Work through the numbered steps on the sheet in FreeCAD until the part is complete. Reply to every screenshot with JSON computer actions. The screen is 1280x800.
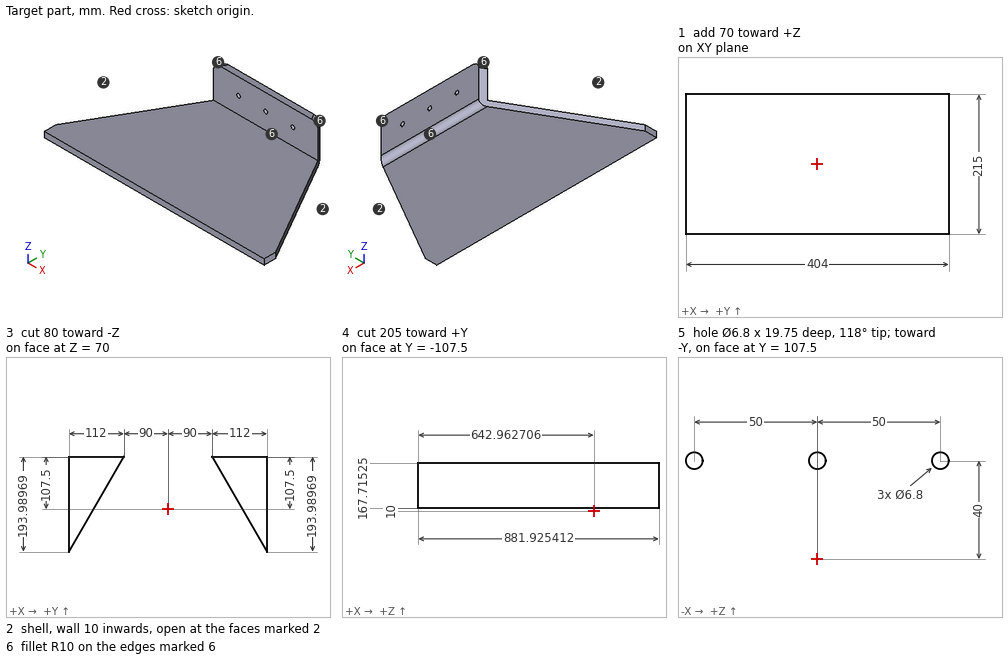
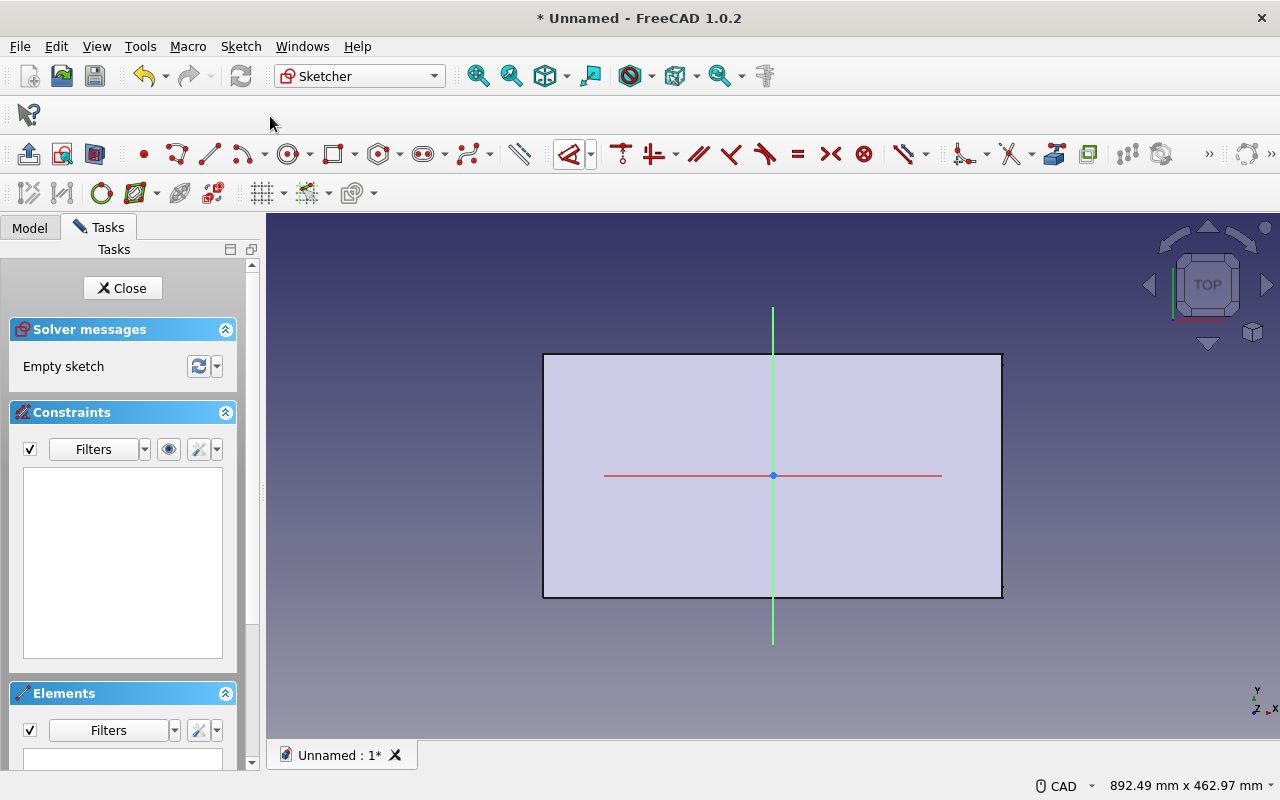
{"action": "left_click", "coordinate": [177, 154]}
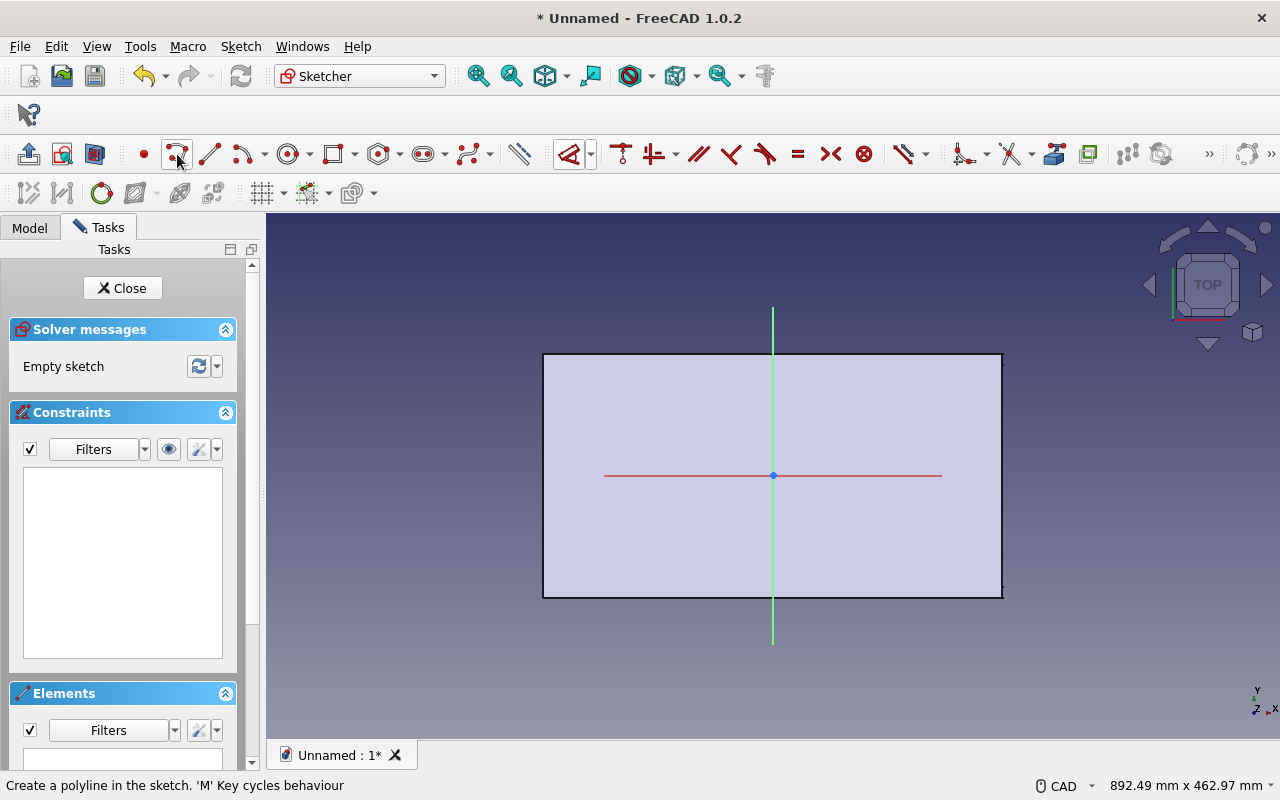
{"action": "left_click", "coordinate": [671, 354]}
{"action": "left_click", "coordinate": [543, 354]}
{"action": "left_click", "coordinate": [543, 574]}
{"action": "left_click", "coordinate": [671, 355]}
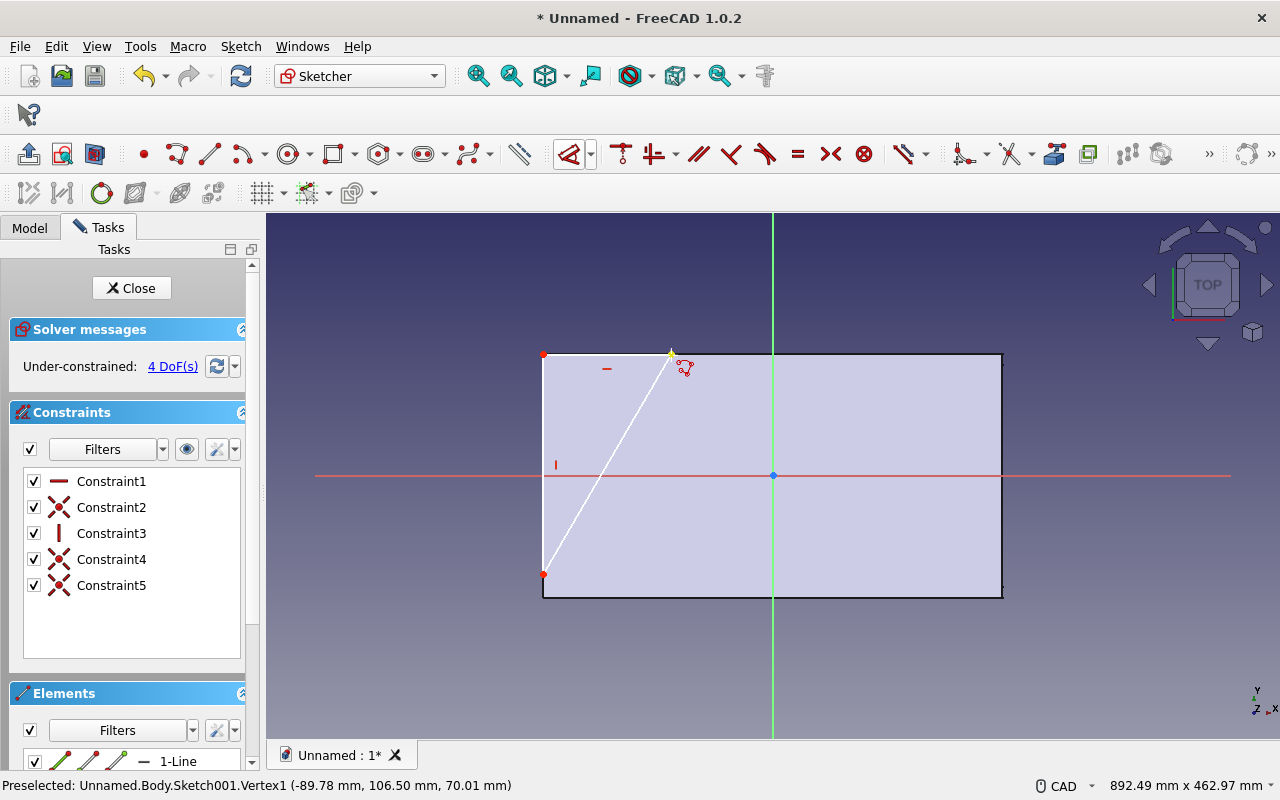
{"action": "left_click", "coordinate": [875, 354]}
{"action": "left_click", "coordinate": [1003, 574]}
{"action": "left_click", "coordinate": [1003, 354]}
{"action": "left_click", "coordinate": [875, 355]}
{"action": "key", "text": "Escape"}
{"action": "key", "text": "Escape"}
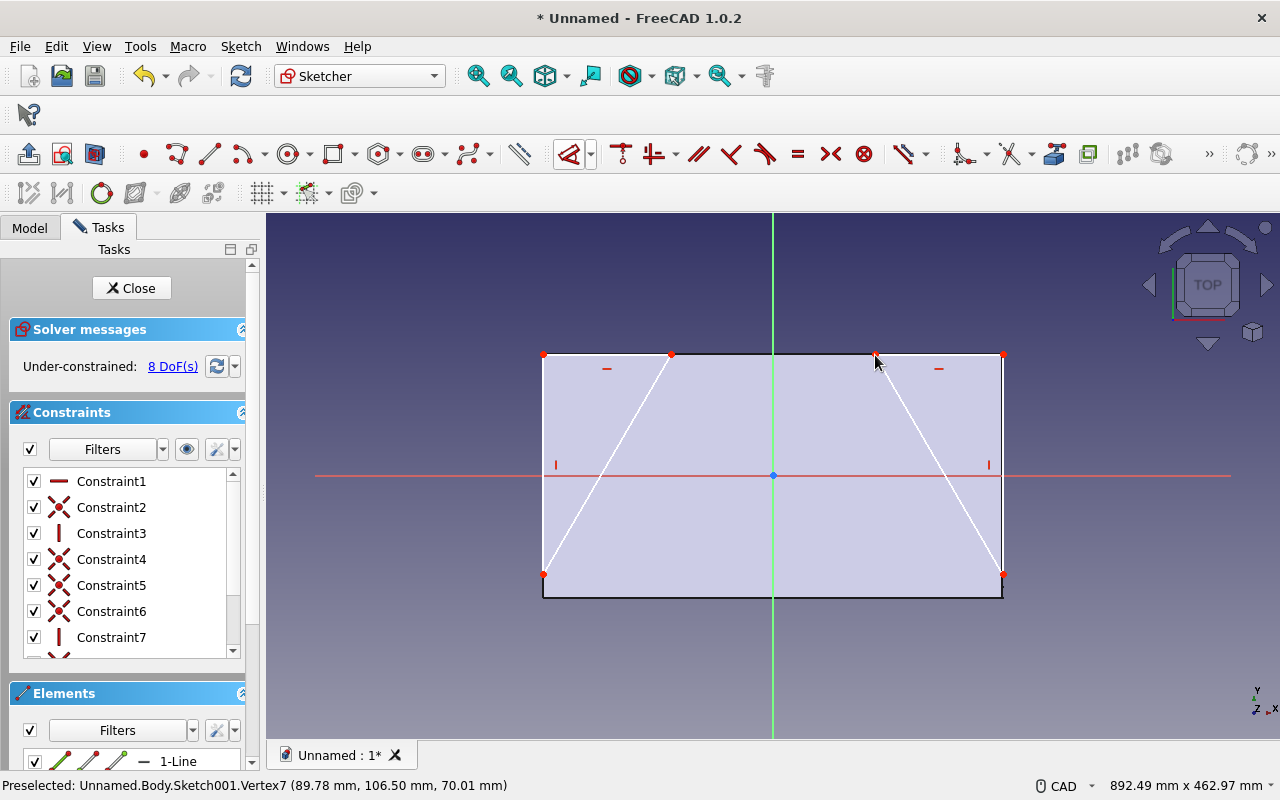
{"action": "left_click", "coordinate": [633, 355]}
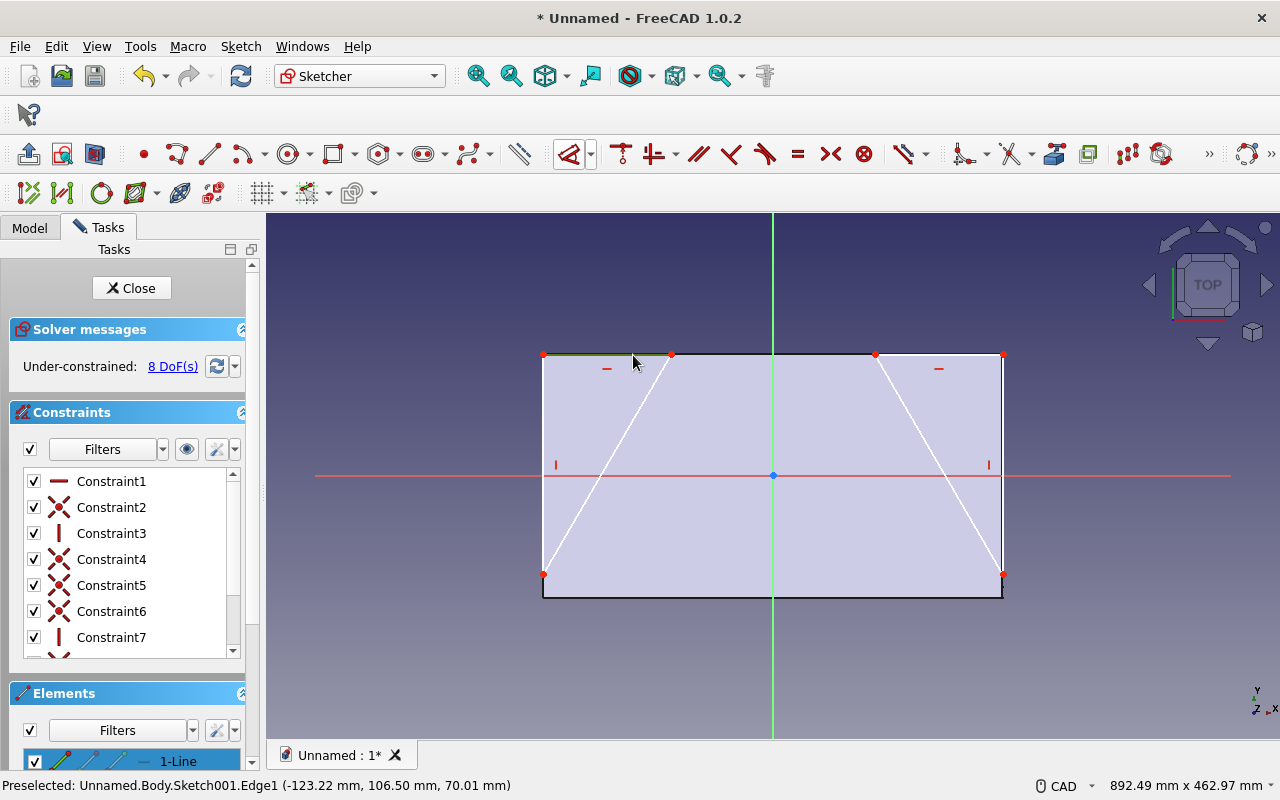
{"action": "left_click", "coordinate": [590, 154]}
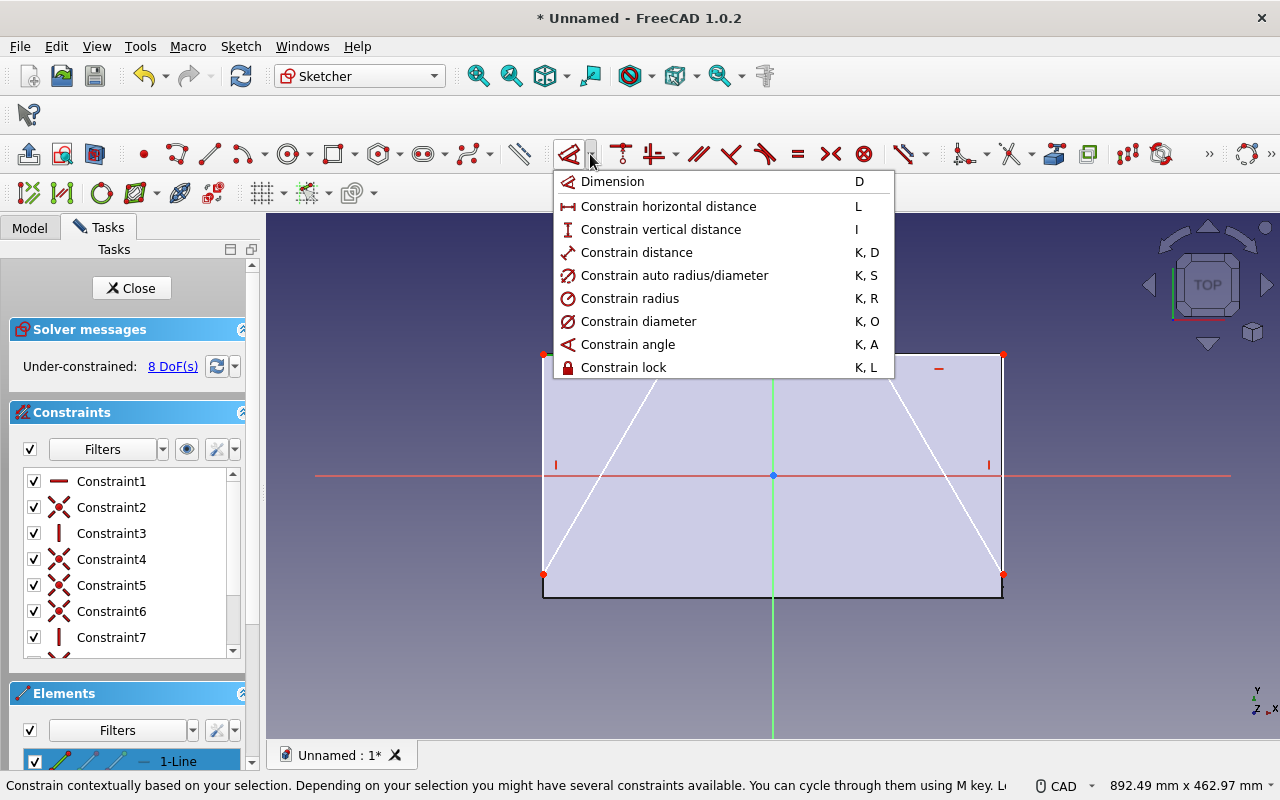
{"action": "left_click", "coordinate": [724, 206]}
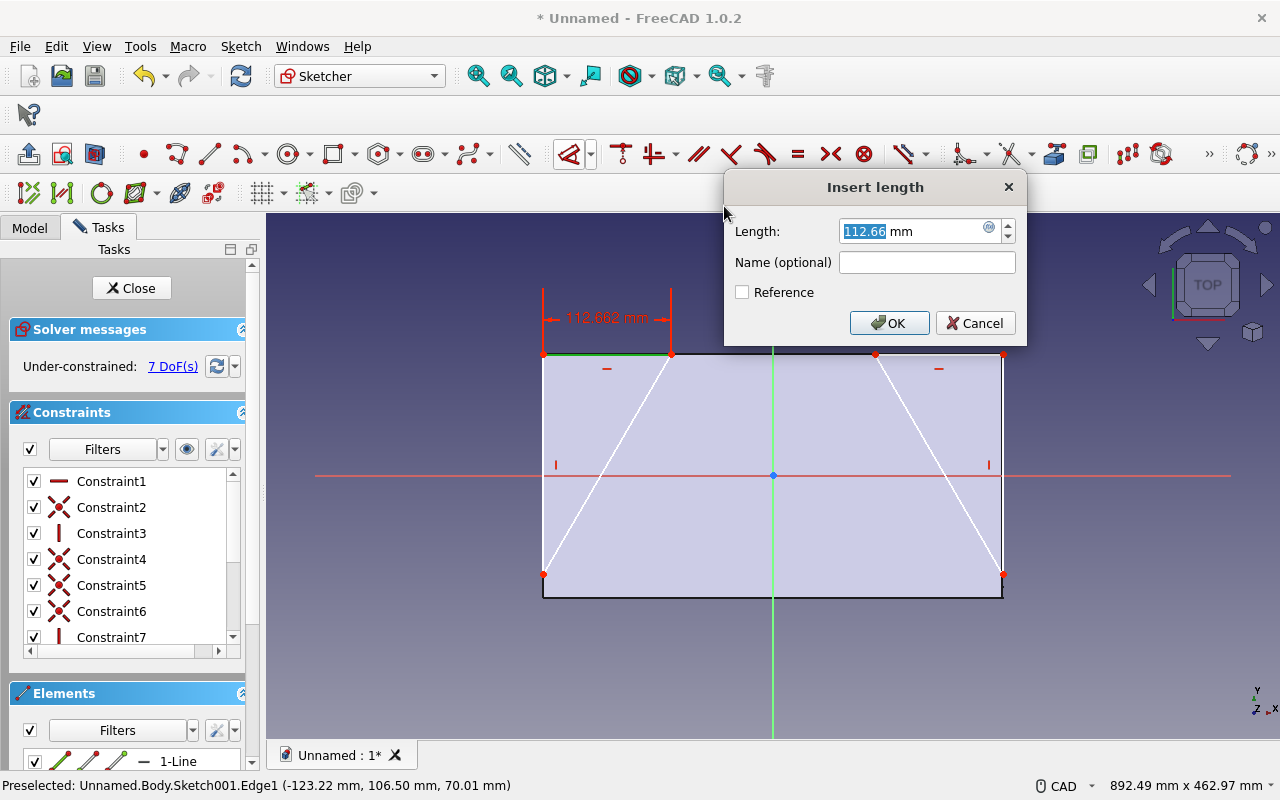
{"action": "type", "text": "112"}
{"action": "key", "text": "Return"}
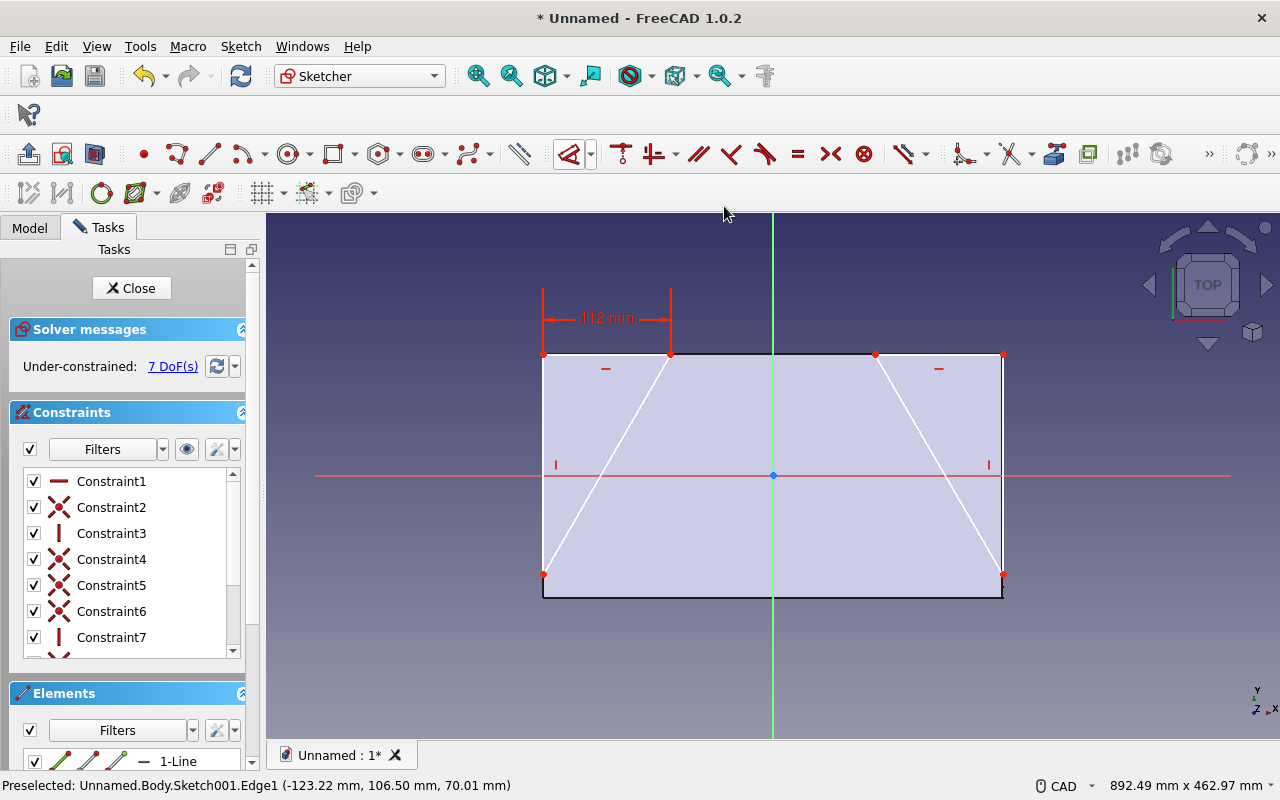
{"action": "left_click", "coordinate": [965, 355]}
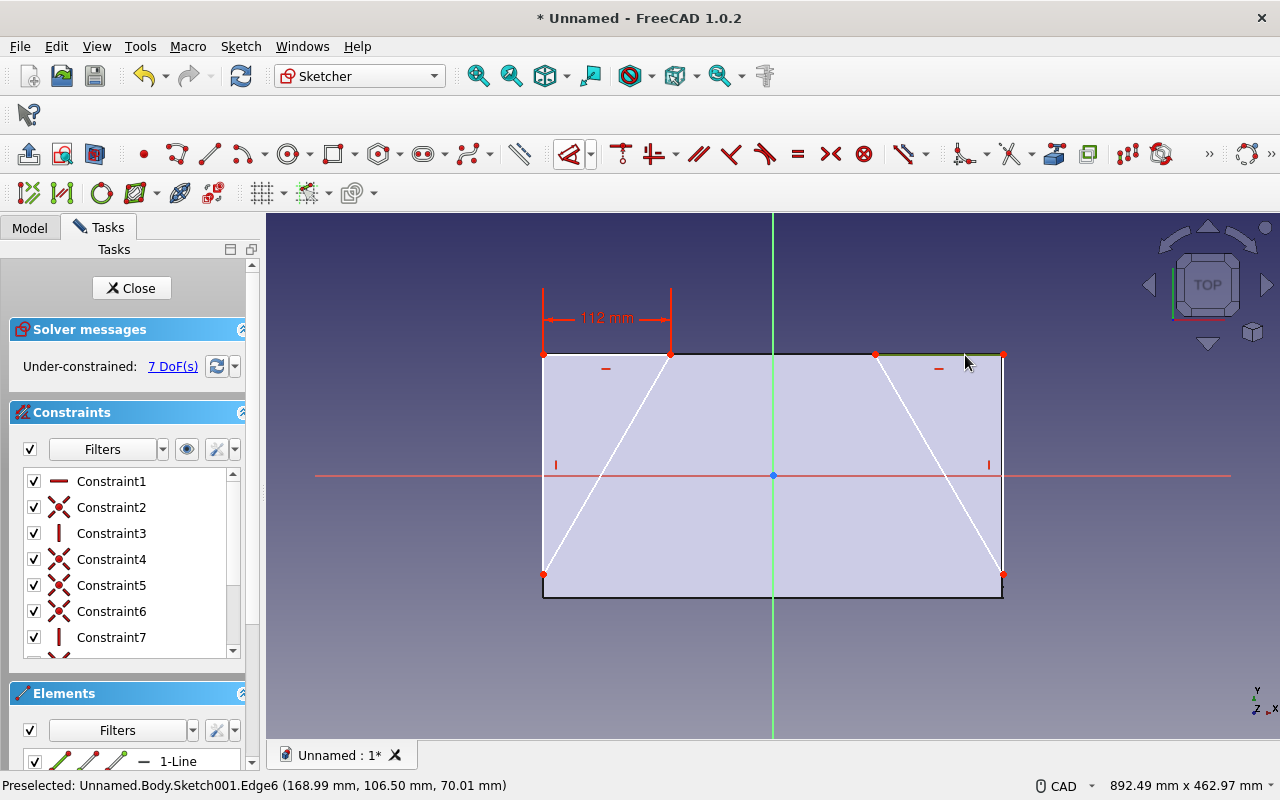
{"action": "left_click", "coordinate": [590, 154]}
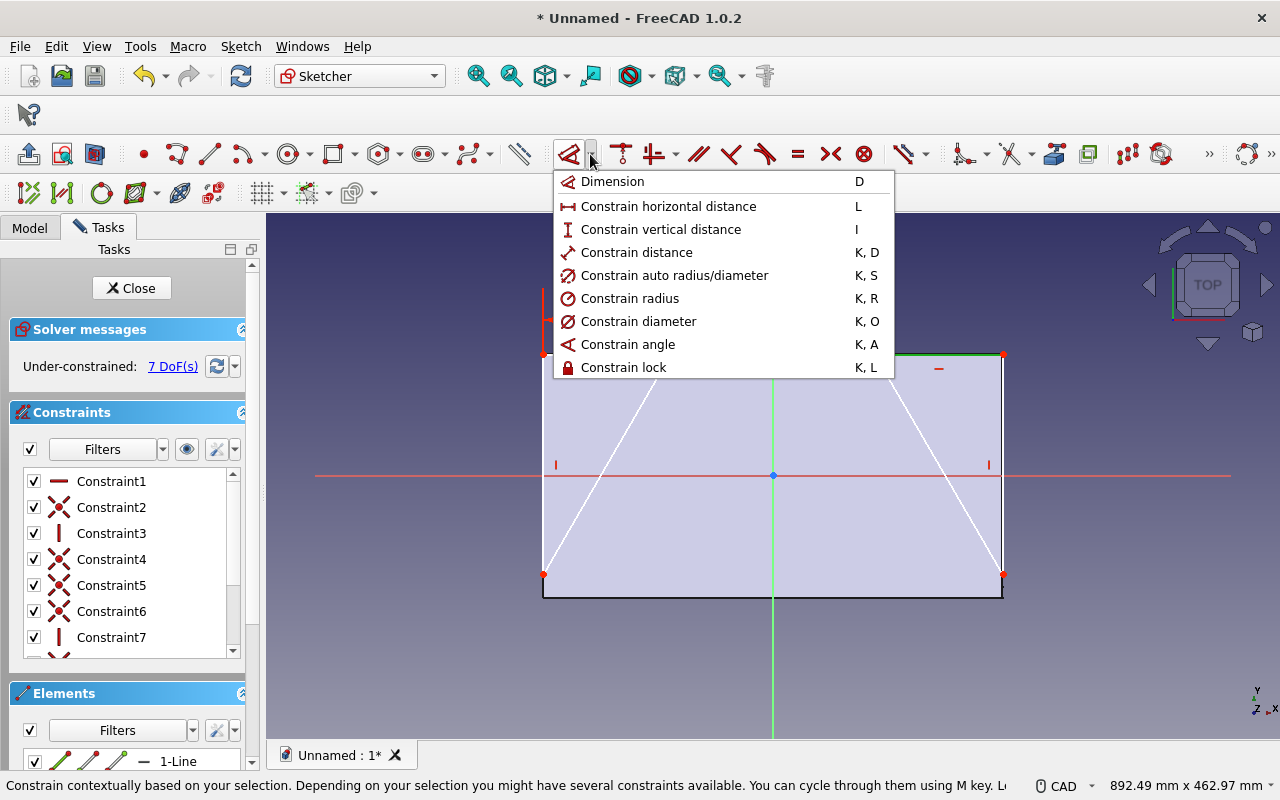
{"action": "left_click", "coordinate": [724, 206]}